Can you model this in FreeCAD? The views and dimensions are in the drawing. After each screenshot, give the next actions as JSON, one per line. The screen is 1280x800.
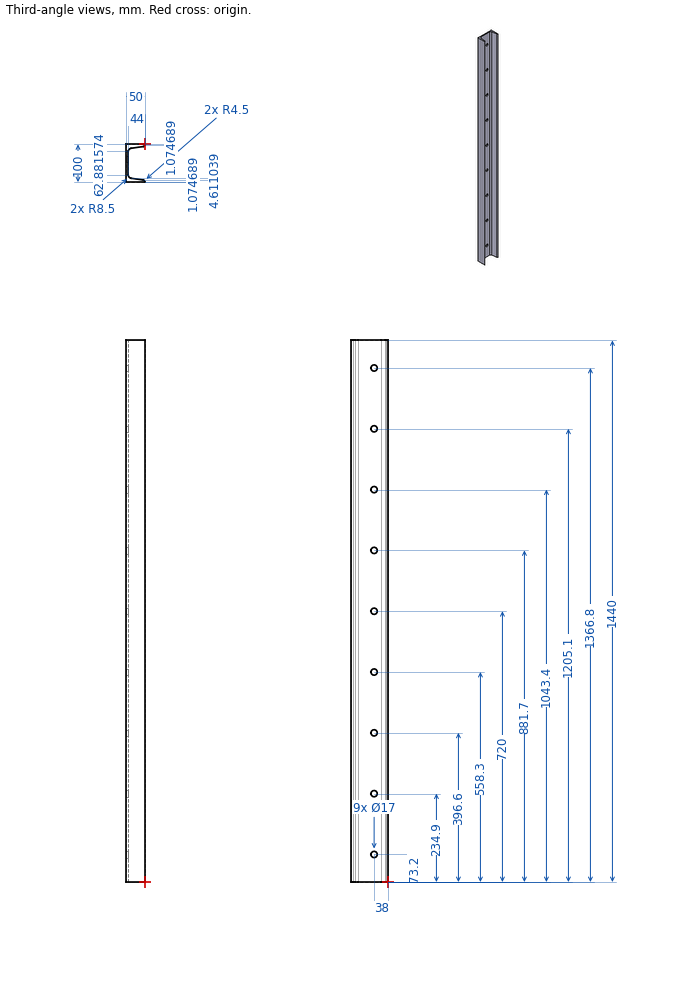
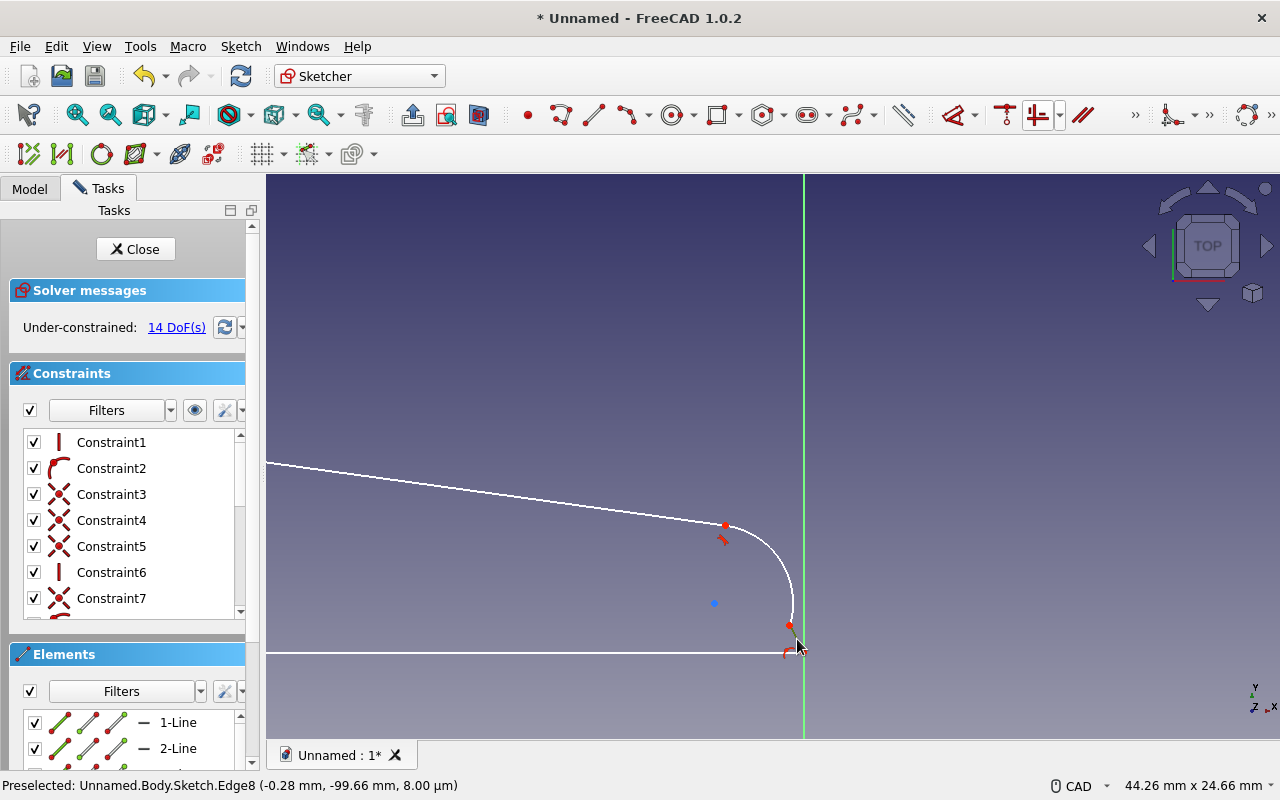
{"action": "left_click", "coordinate": [791, 585]}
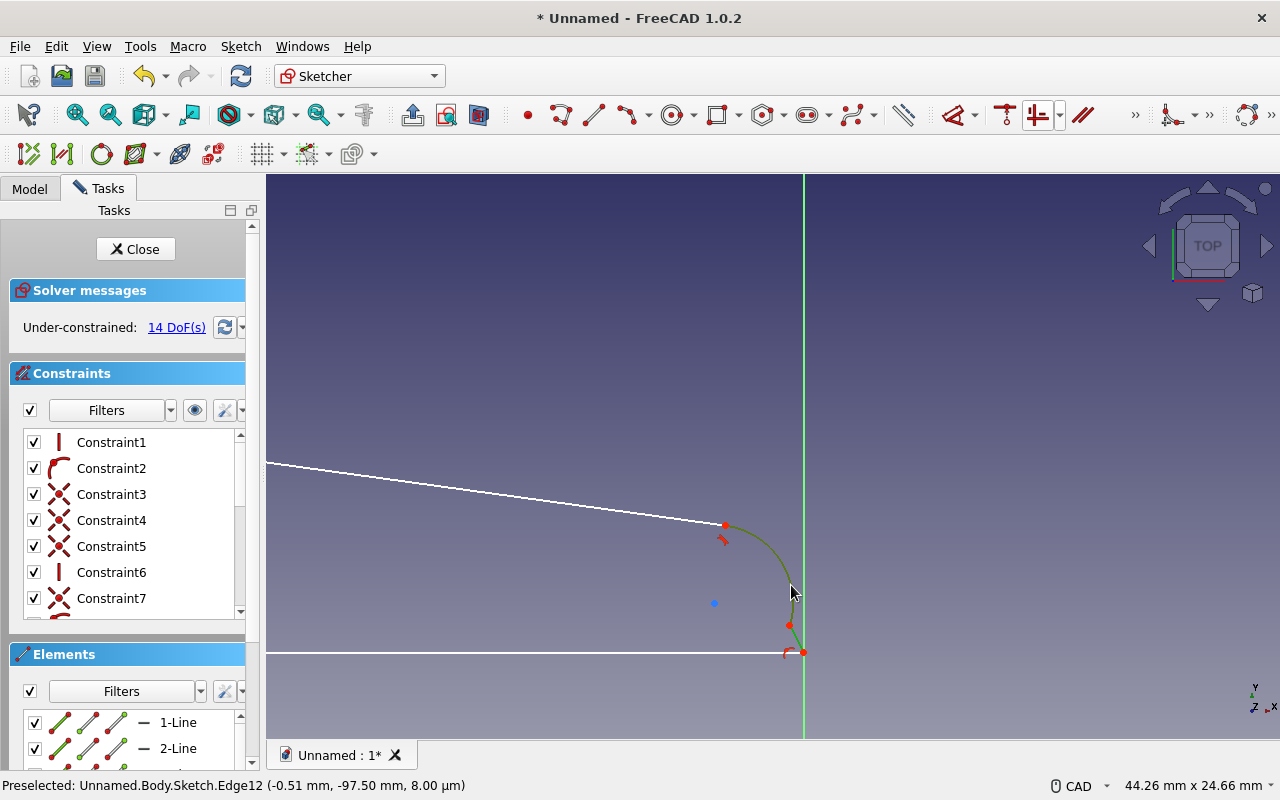
{"action": "key", "text": "t"}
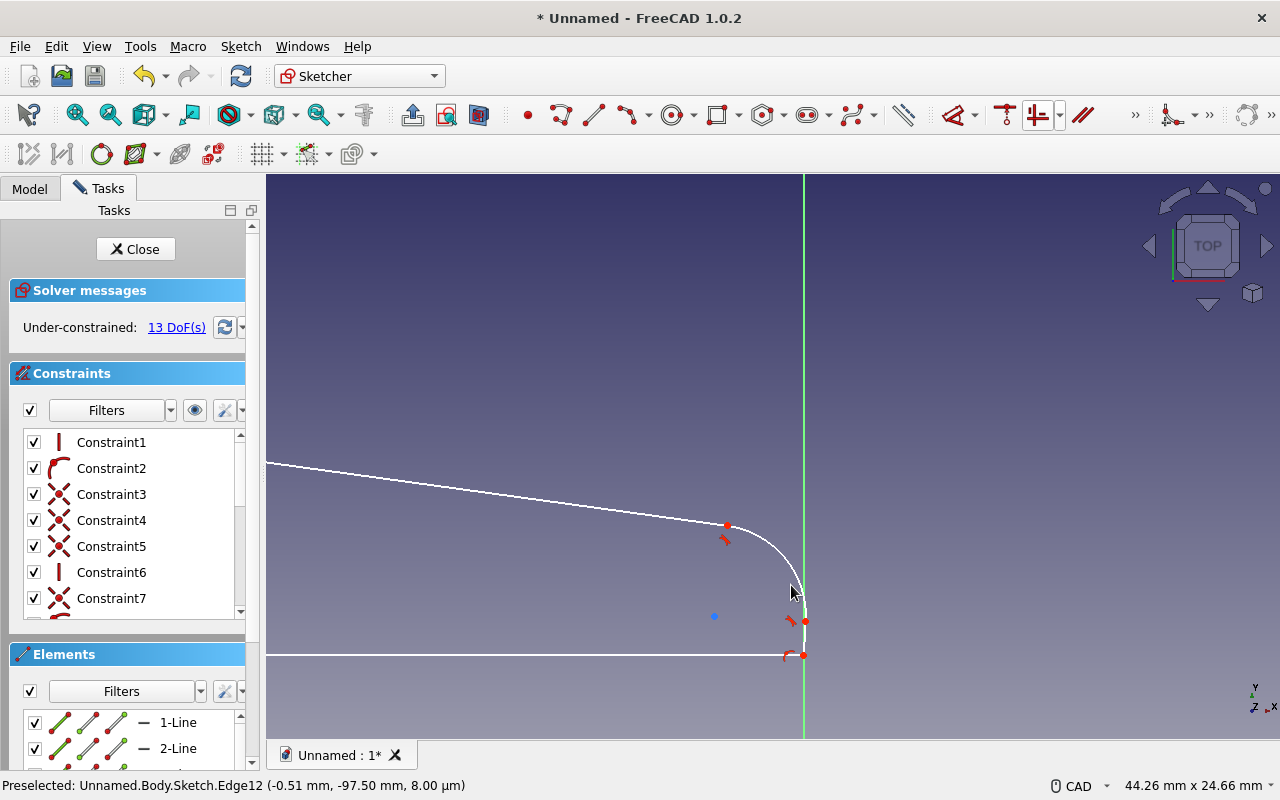
{"action": "scroll", "coordinate": [798, 646], "scroll_direction": "down", "scroll_amount": 9}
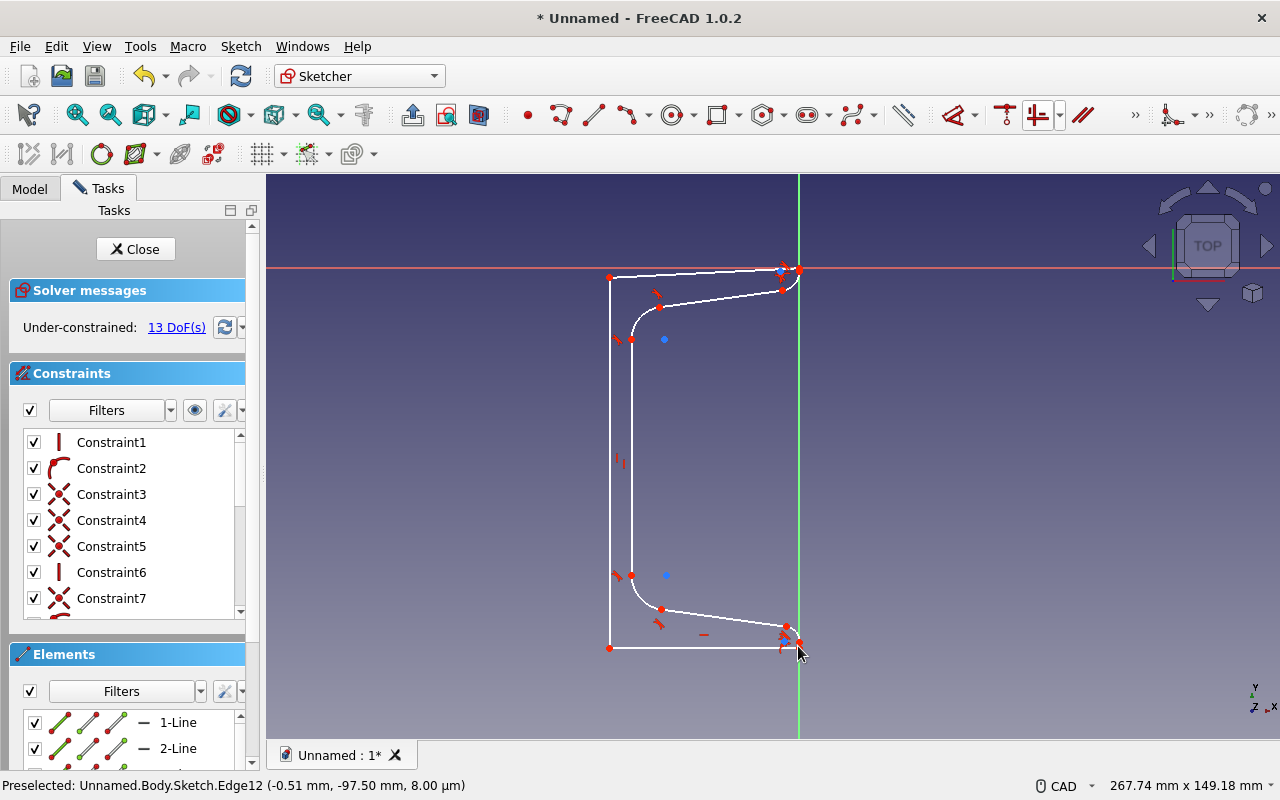
{"action": "scroll", "coordinate": [743, 271], "scroll_direction": "up", "scroll_amount": 8}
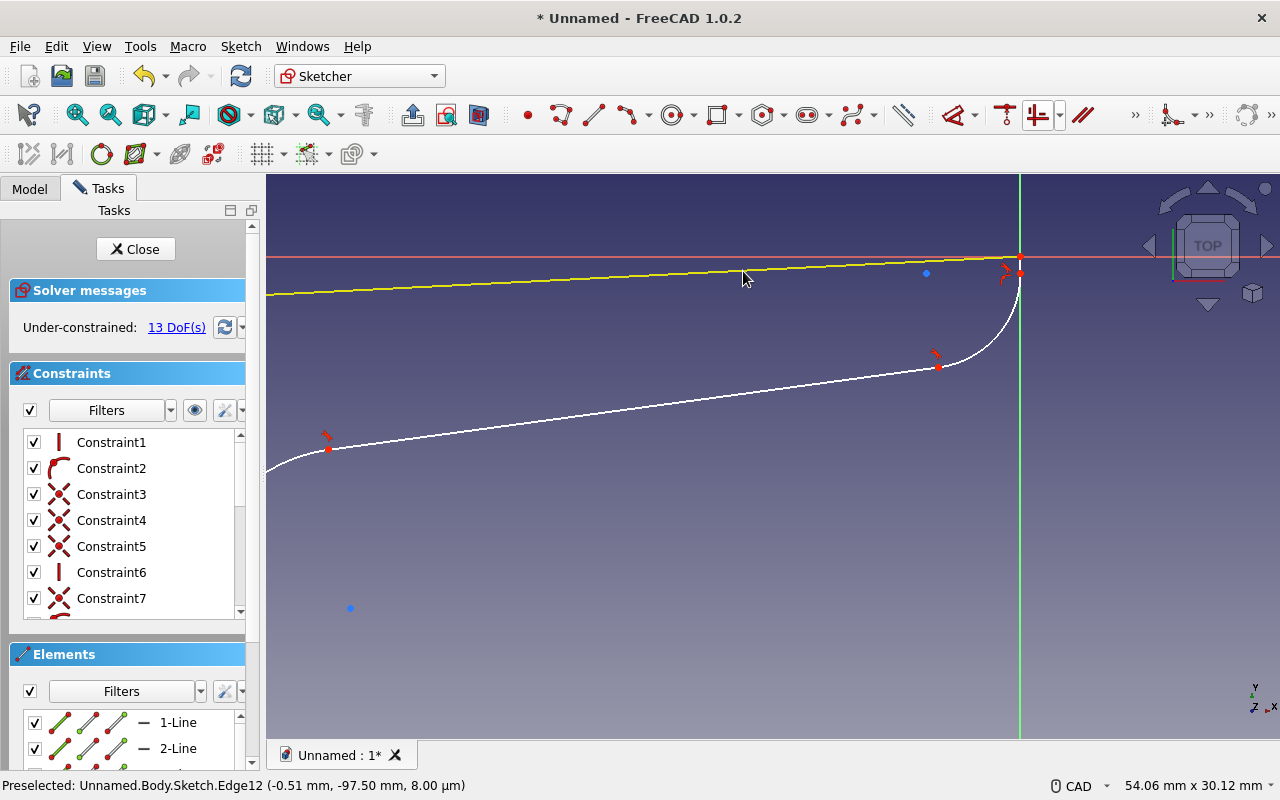
{"action": "left_click", "coordinate": [739, 271]}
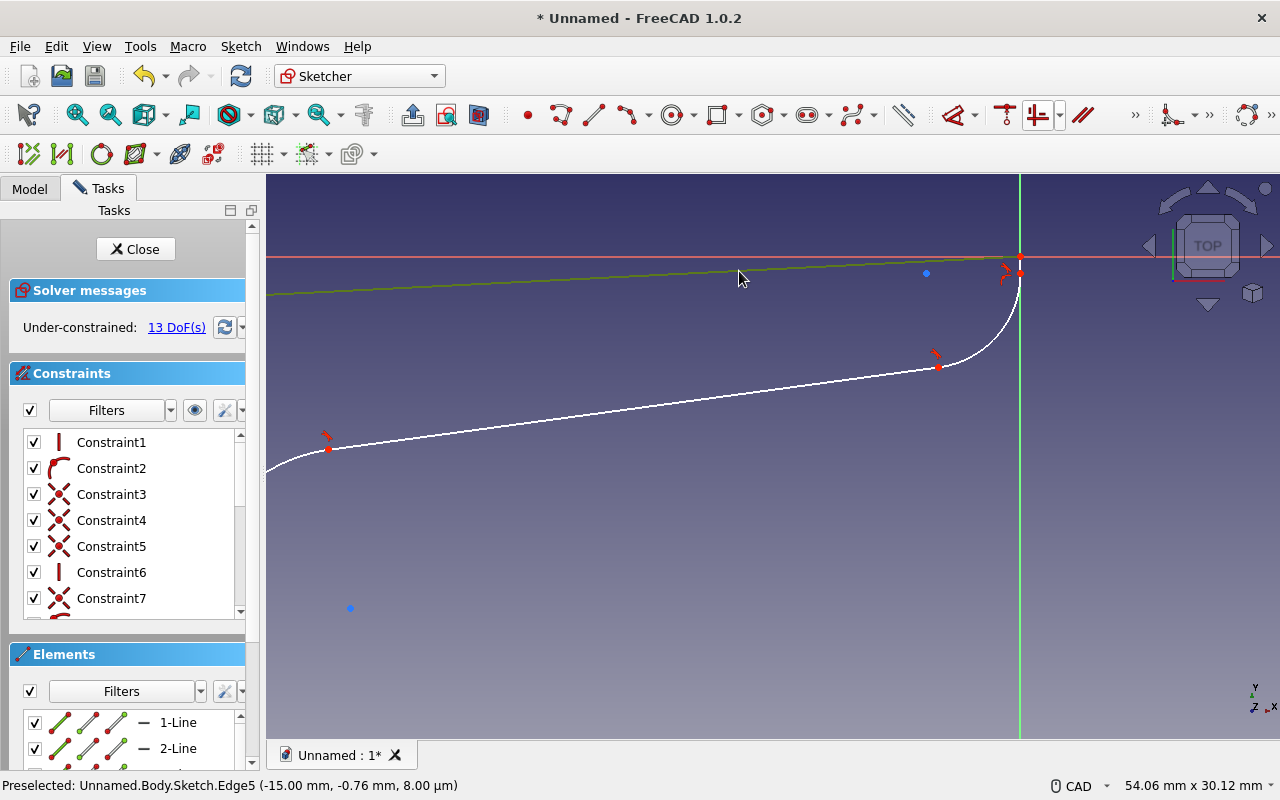
{"action": "key", "text": "h"}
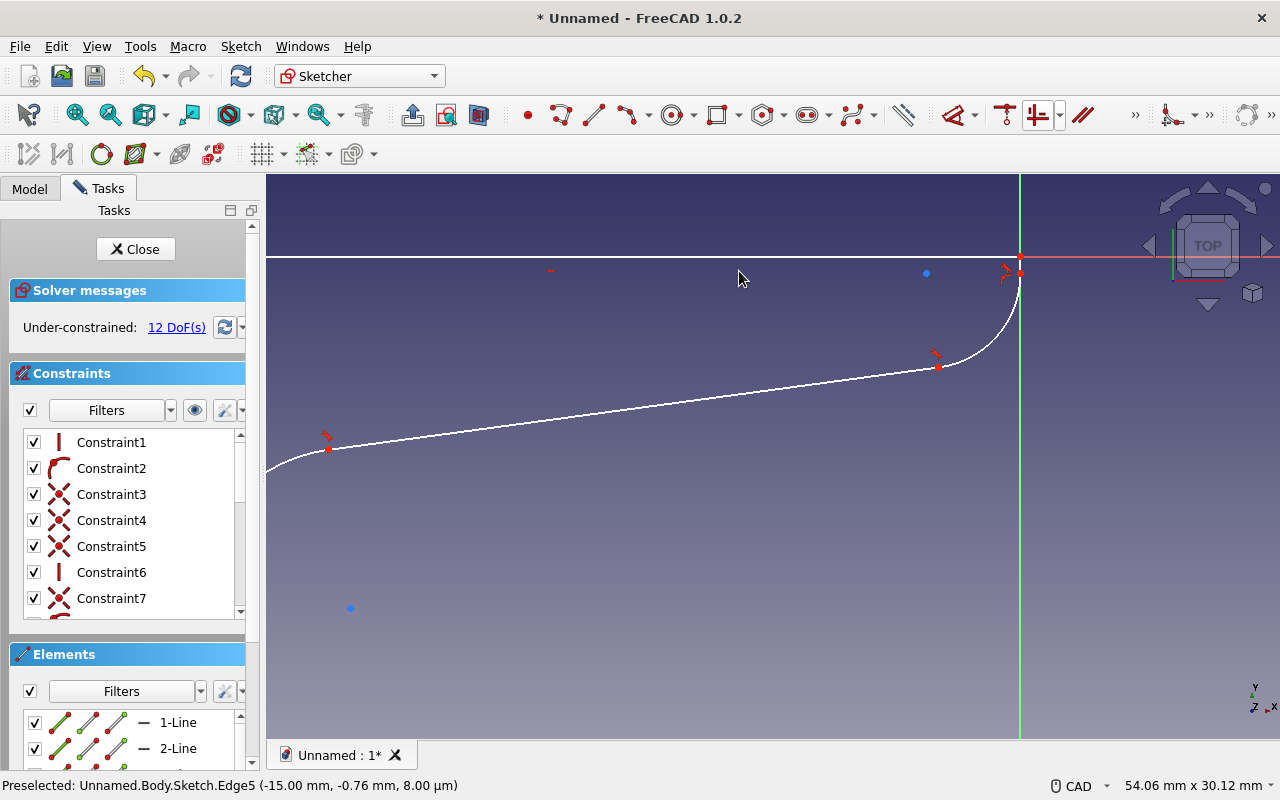
{"action": "scroll", "coordinate": [743, 270], "scroll_direction": "down", "scroll_amount": 8}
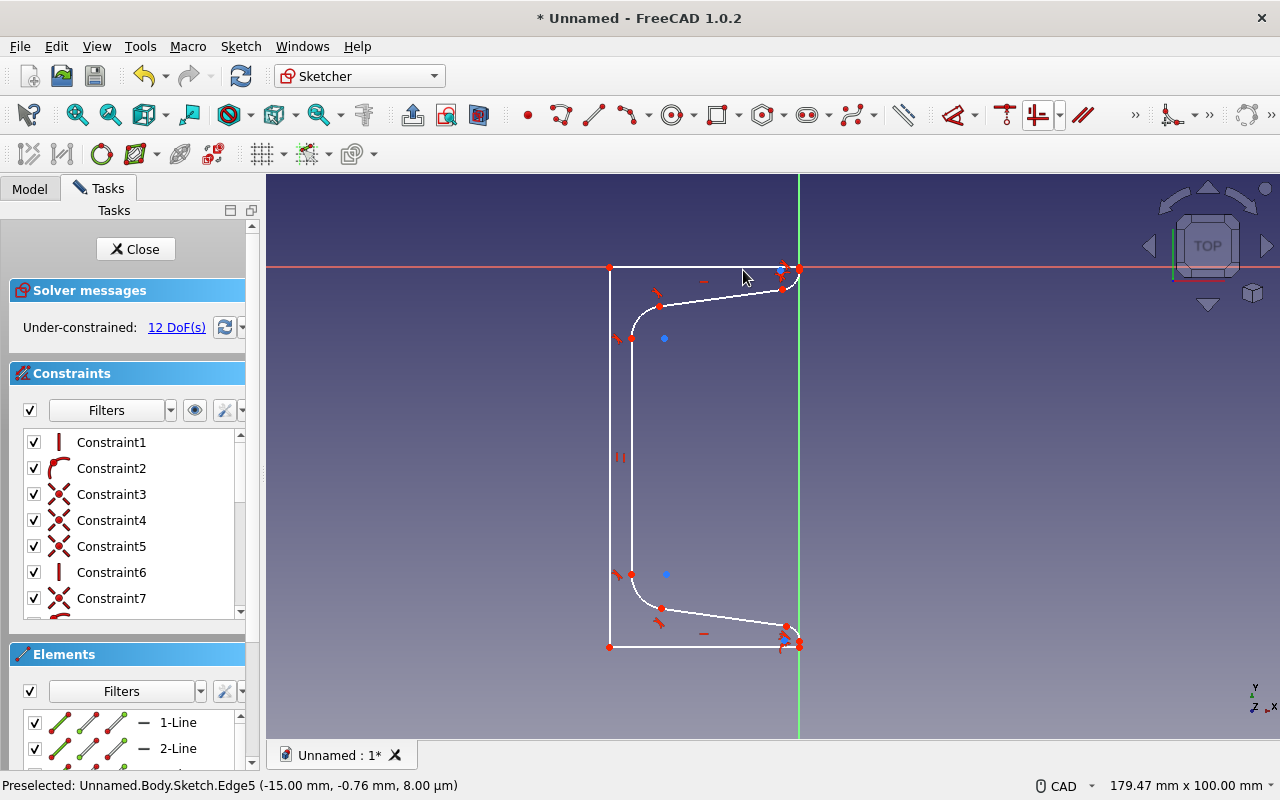
{"action": "scroll", "coordinate": [800, 645], "scroll_direction": "up", "scroll_amount": 10}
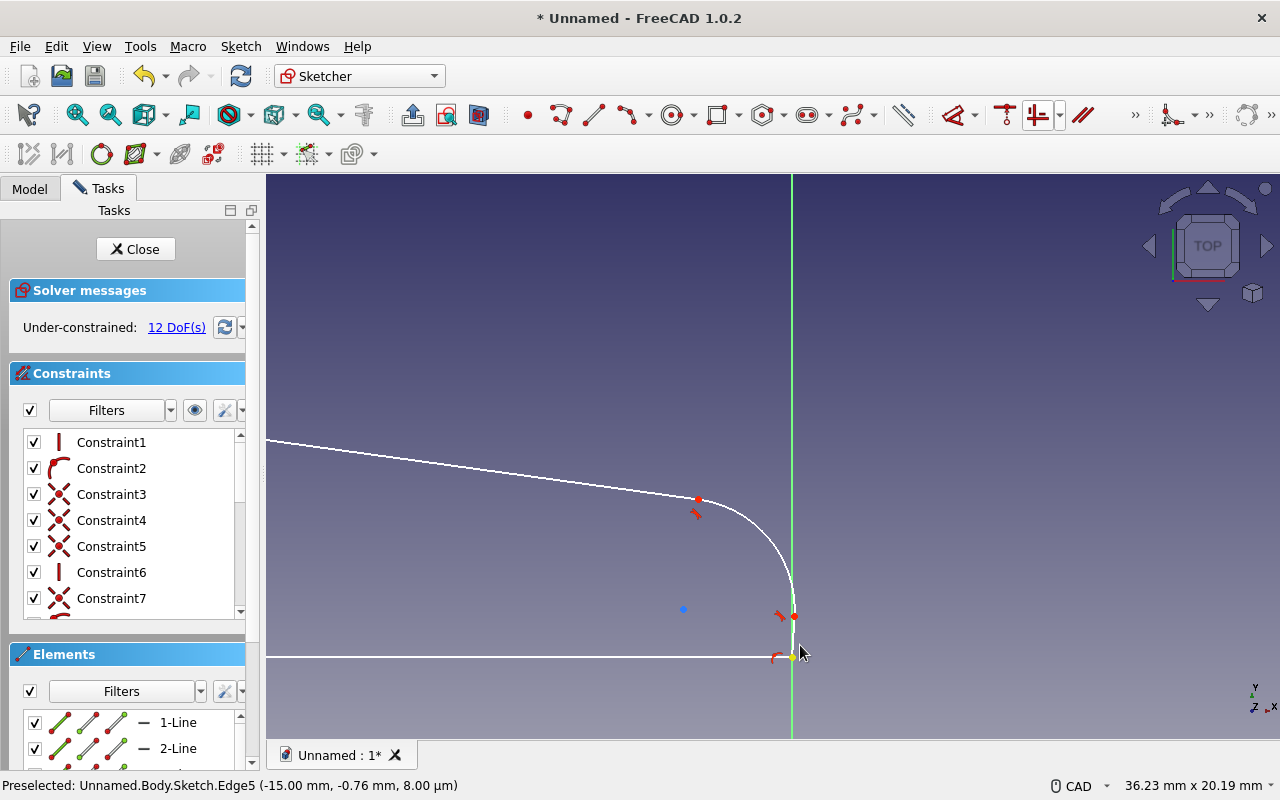
{"action": "left_click", "coordinate": [793, 641]}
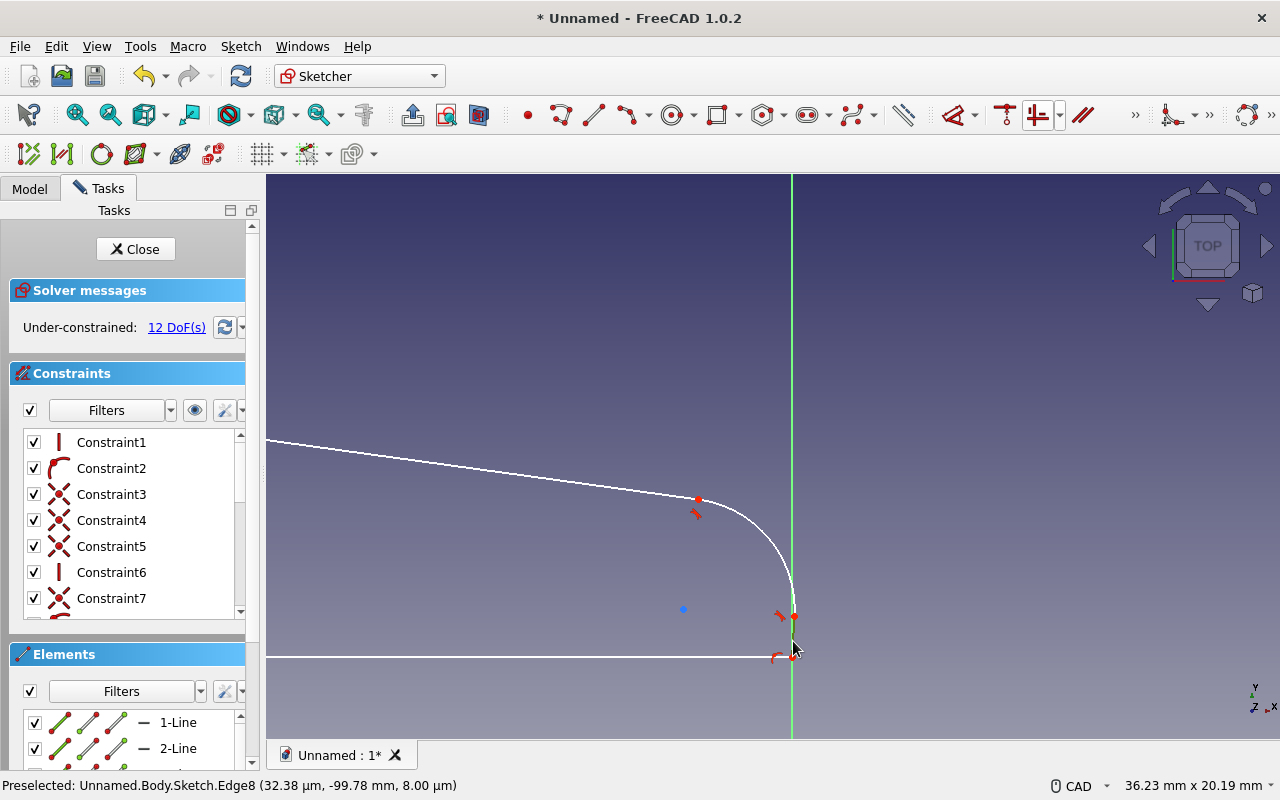
{"action": "key", "text": "v"}